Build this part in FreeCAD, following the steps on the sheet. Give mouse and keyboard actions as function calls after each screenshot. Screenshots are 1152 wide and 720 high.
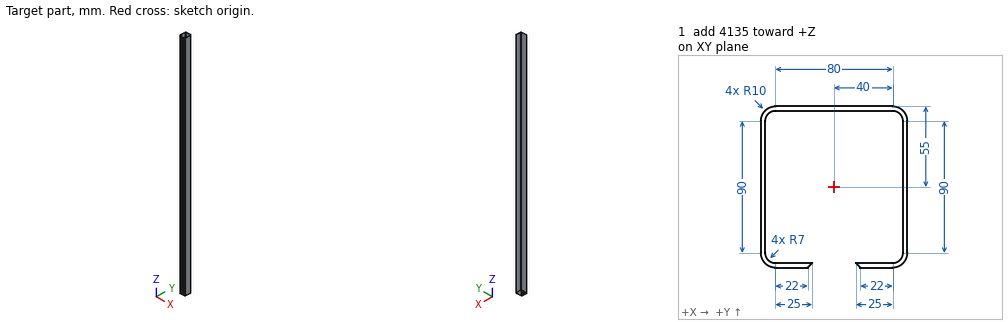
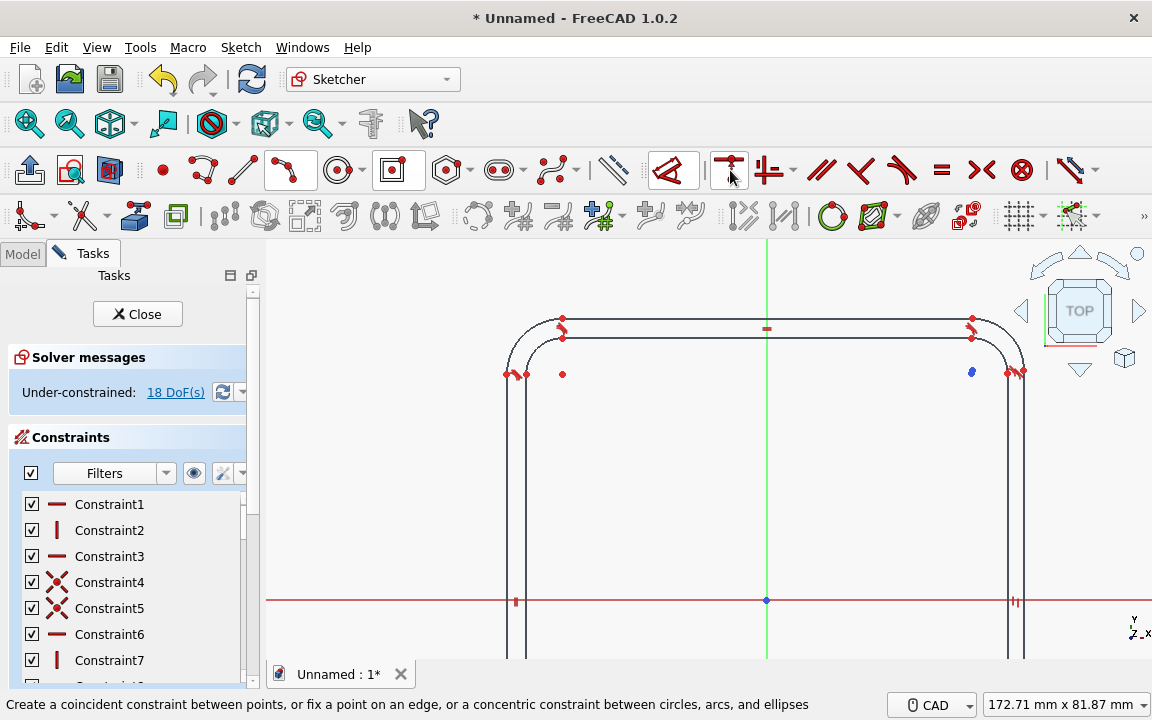
scroll(537, 326, down, 4)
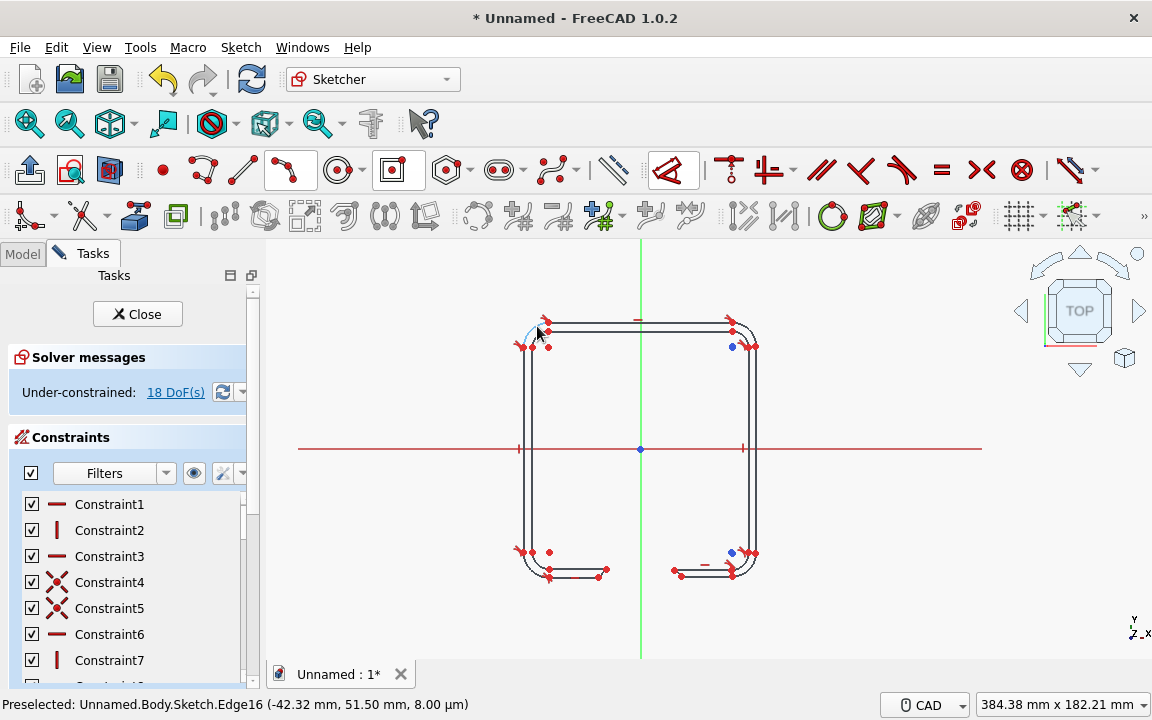
scroll(739, 568, up, 4)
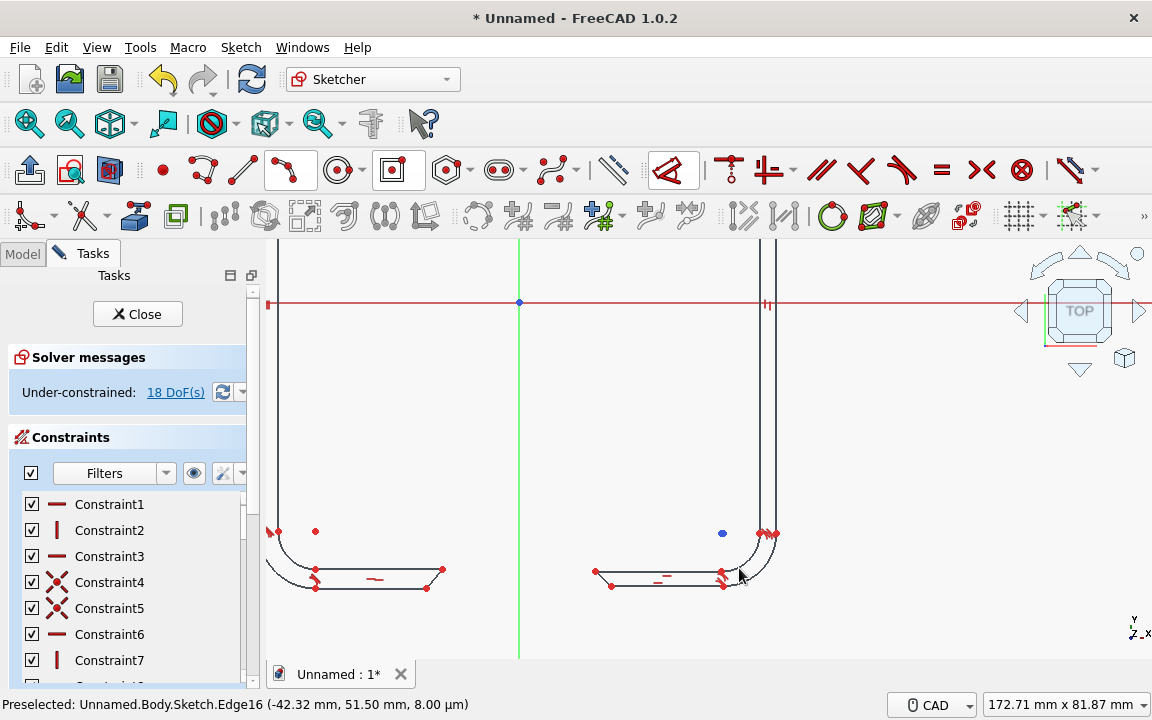
click(739, 567)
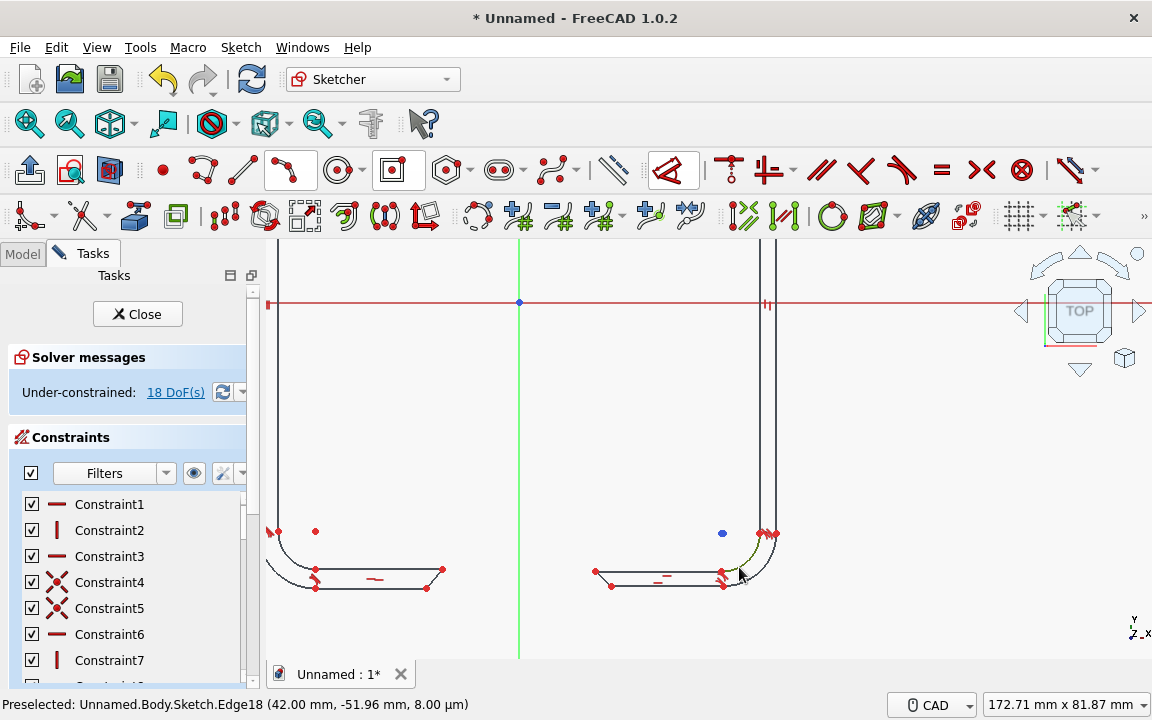
click(748, 580)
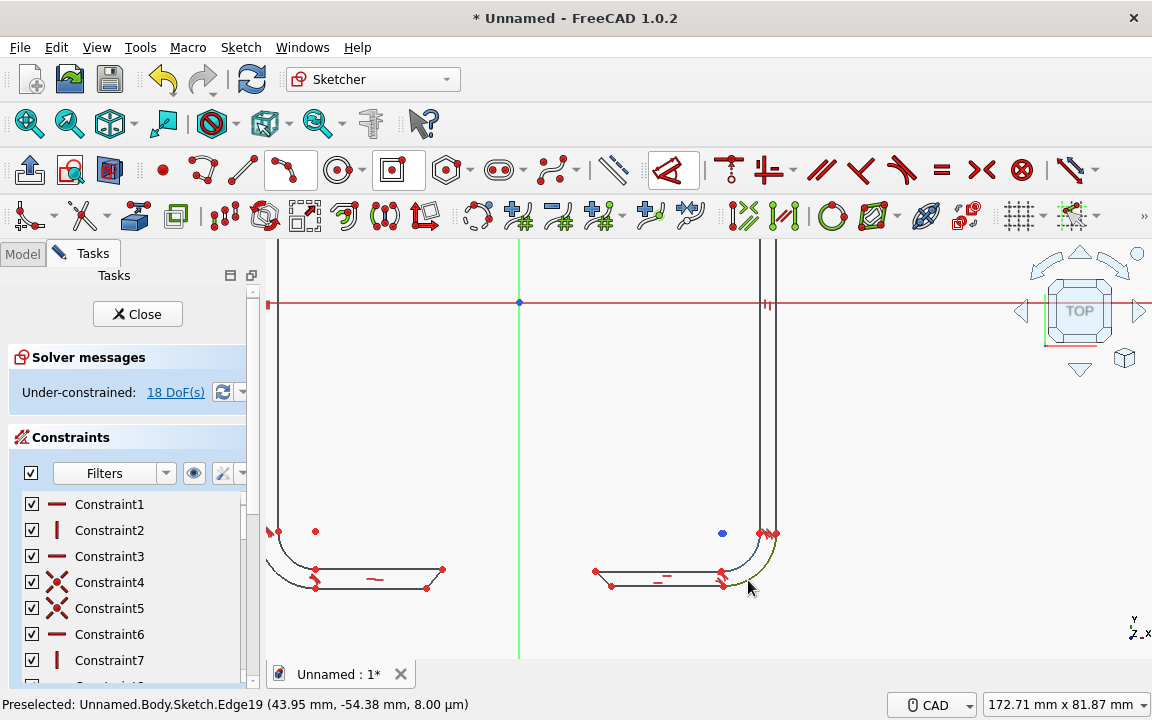
click(730, 170)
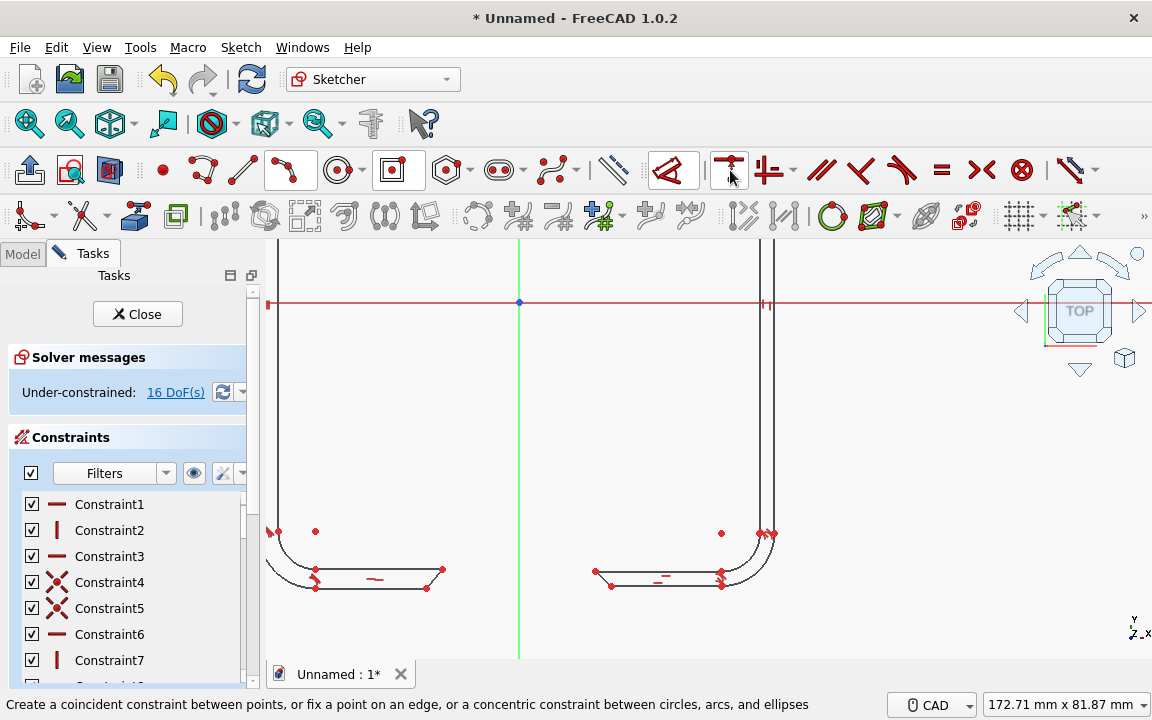
scroll(740, 568, down, 4)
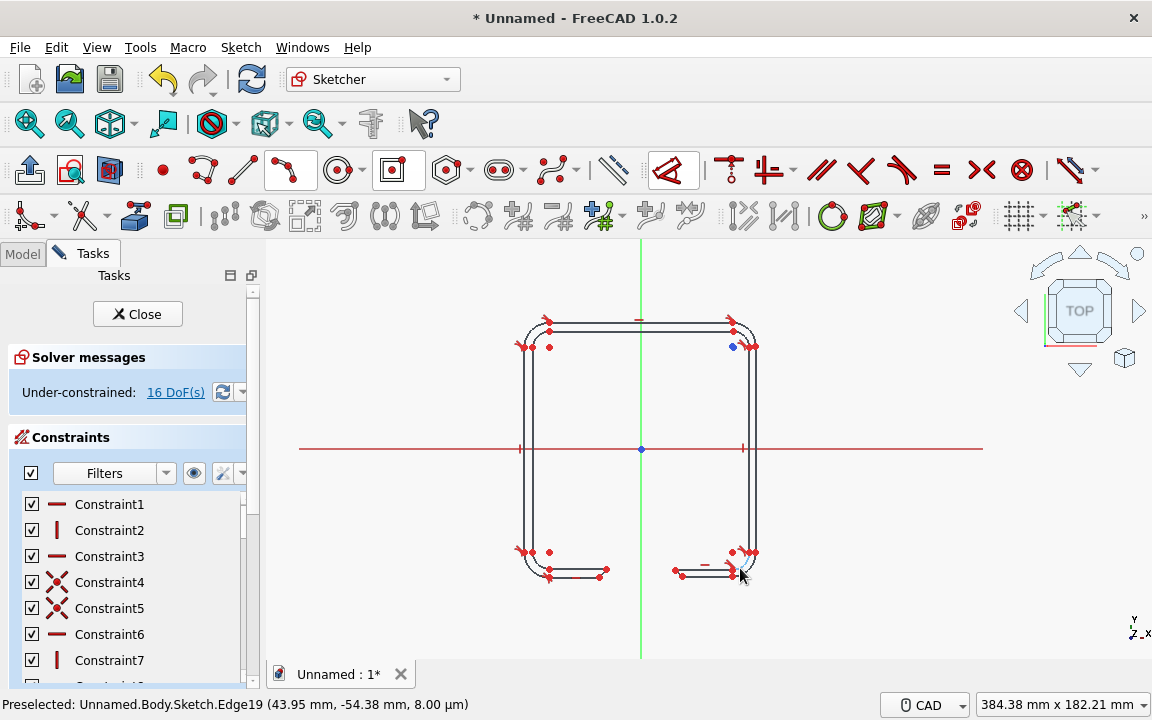
scroll(747, 340, up, 4)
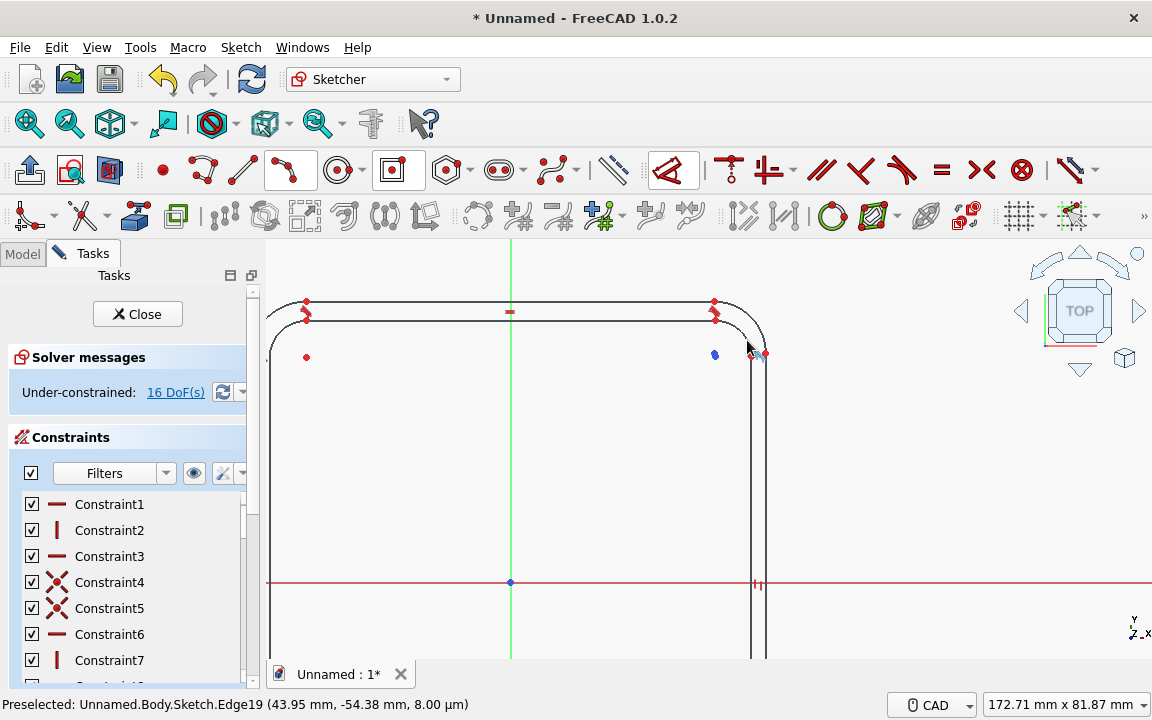
click(747, 341)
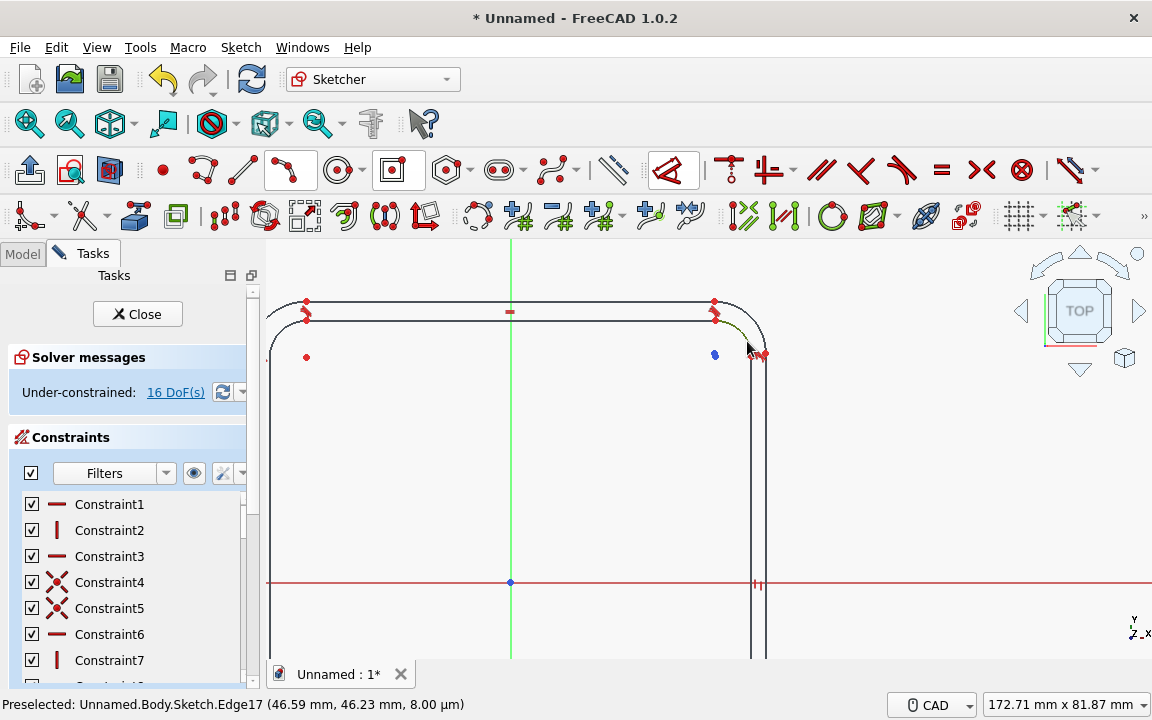
click(760, 330)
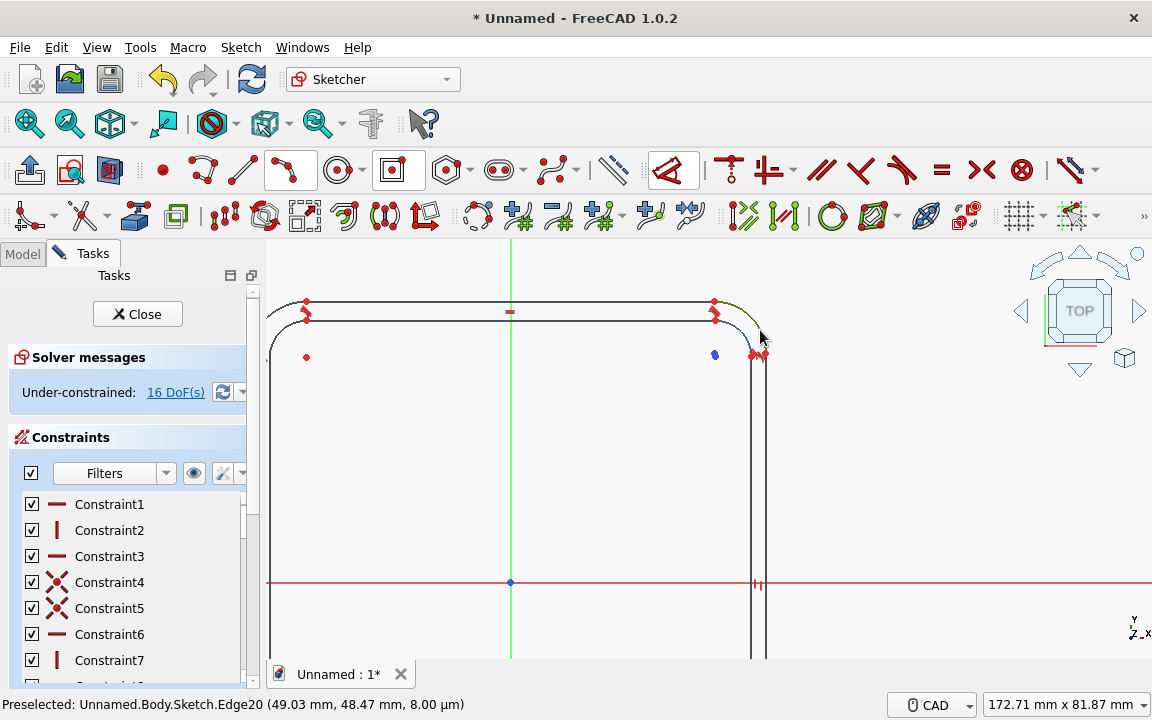
click(730, 170)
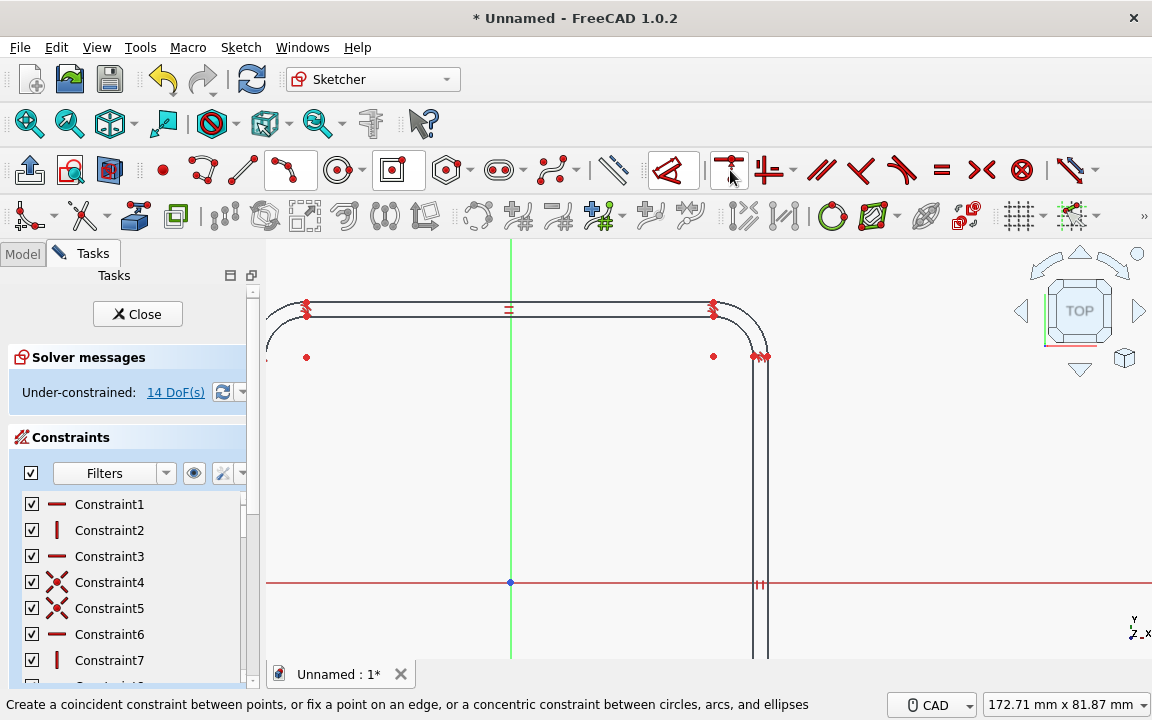
scroll(747, 340, down, 4)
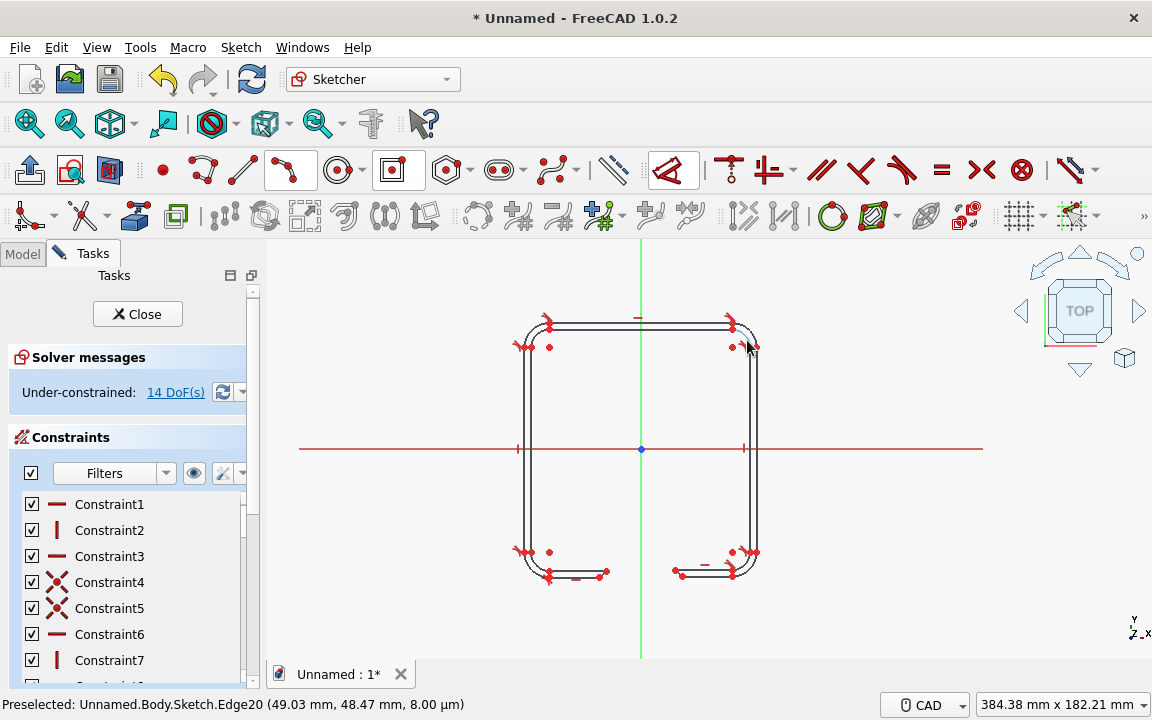
scroll(538, 326, up, 4)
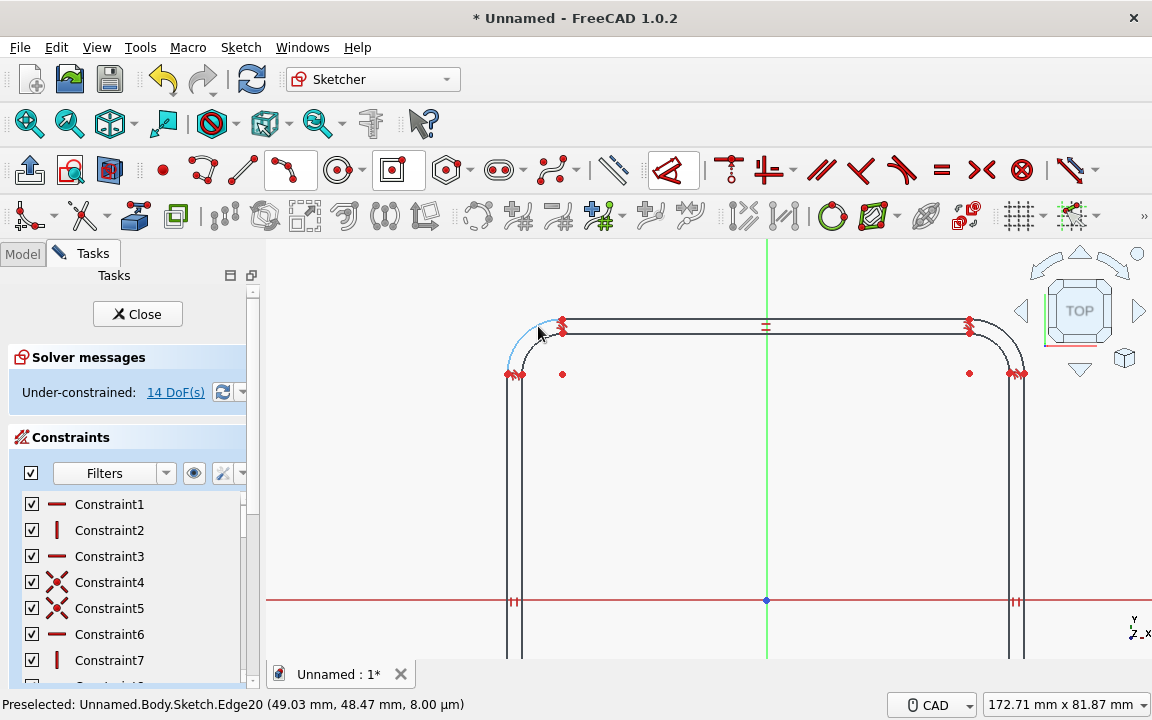
click(538, 325)